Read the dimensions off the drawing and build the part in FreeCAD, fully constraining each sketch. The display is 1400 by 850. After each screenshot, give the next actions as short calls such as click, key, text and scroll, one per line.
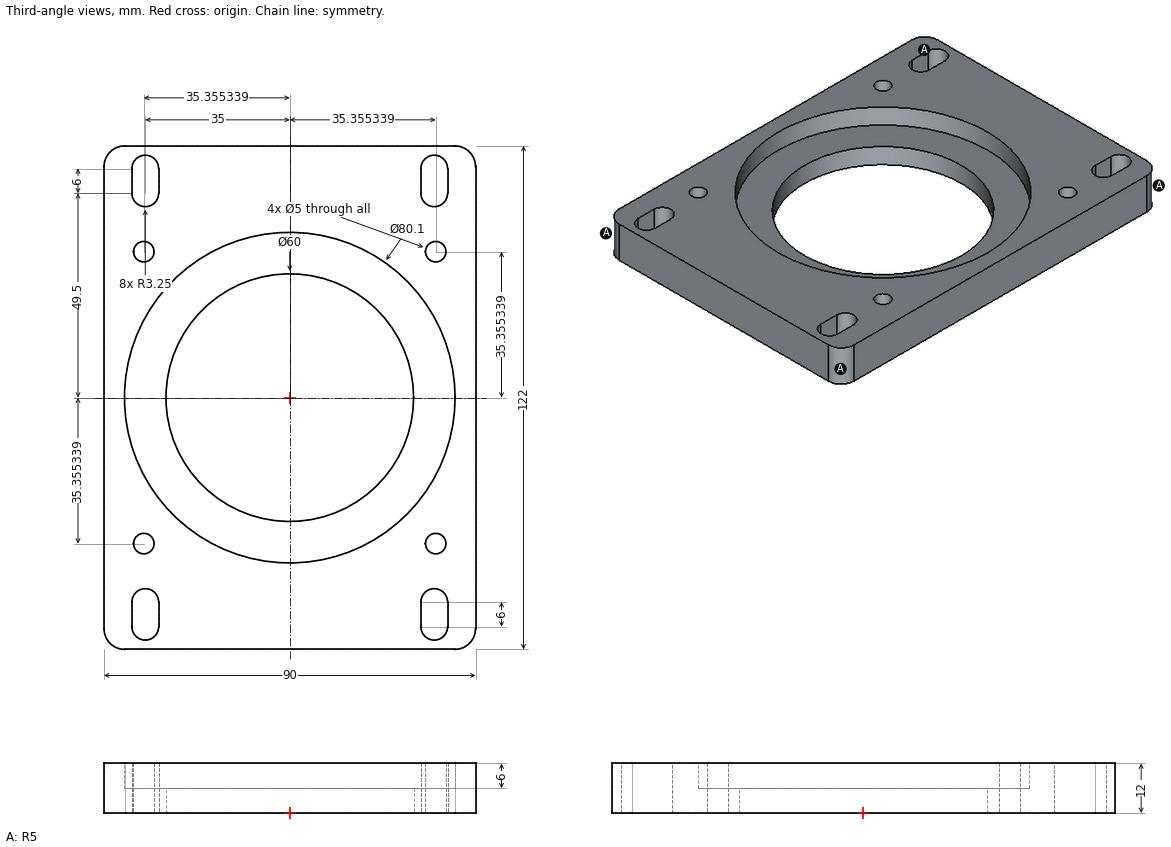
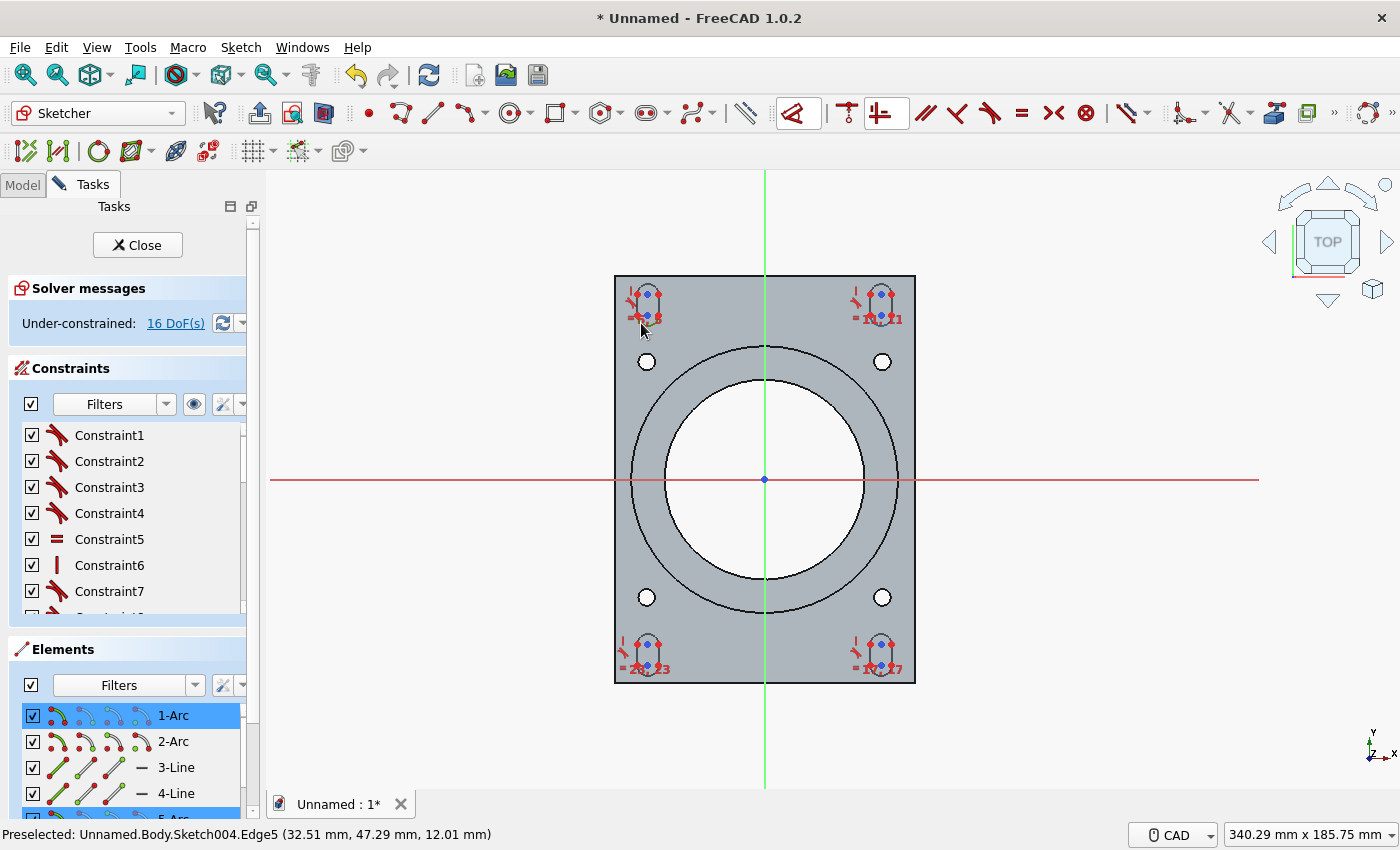
scroll(875, 674, up, 2)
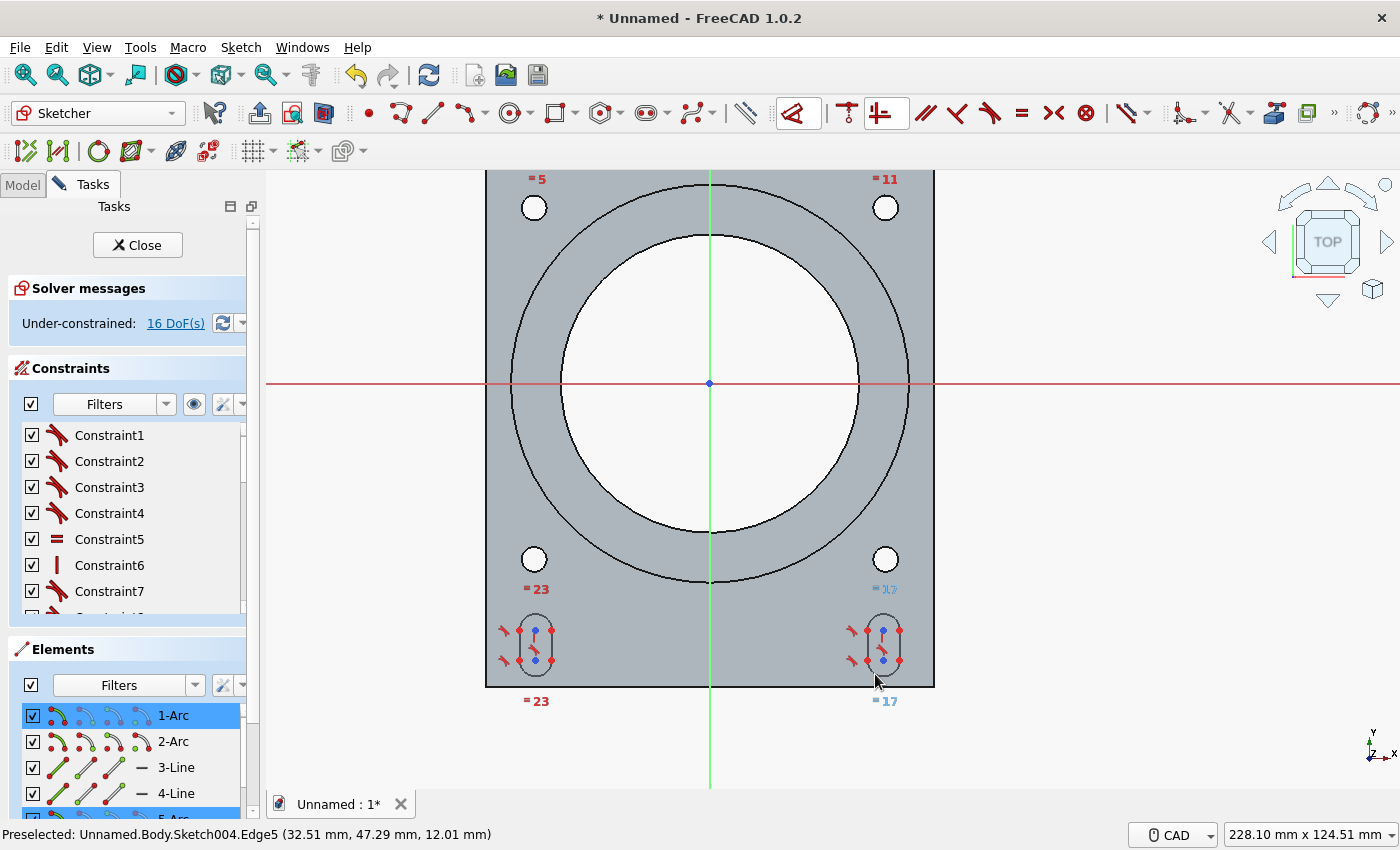
click(874, 673)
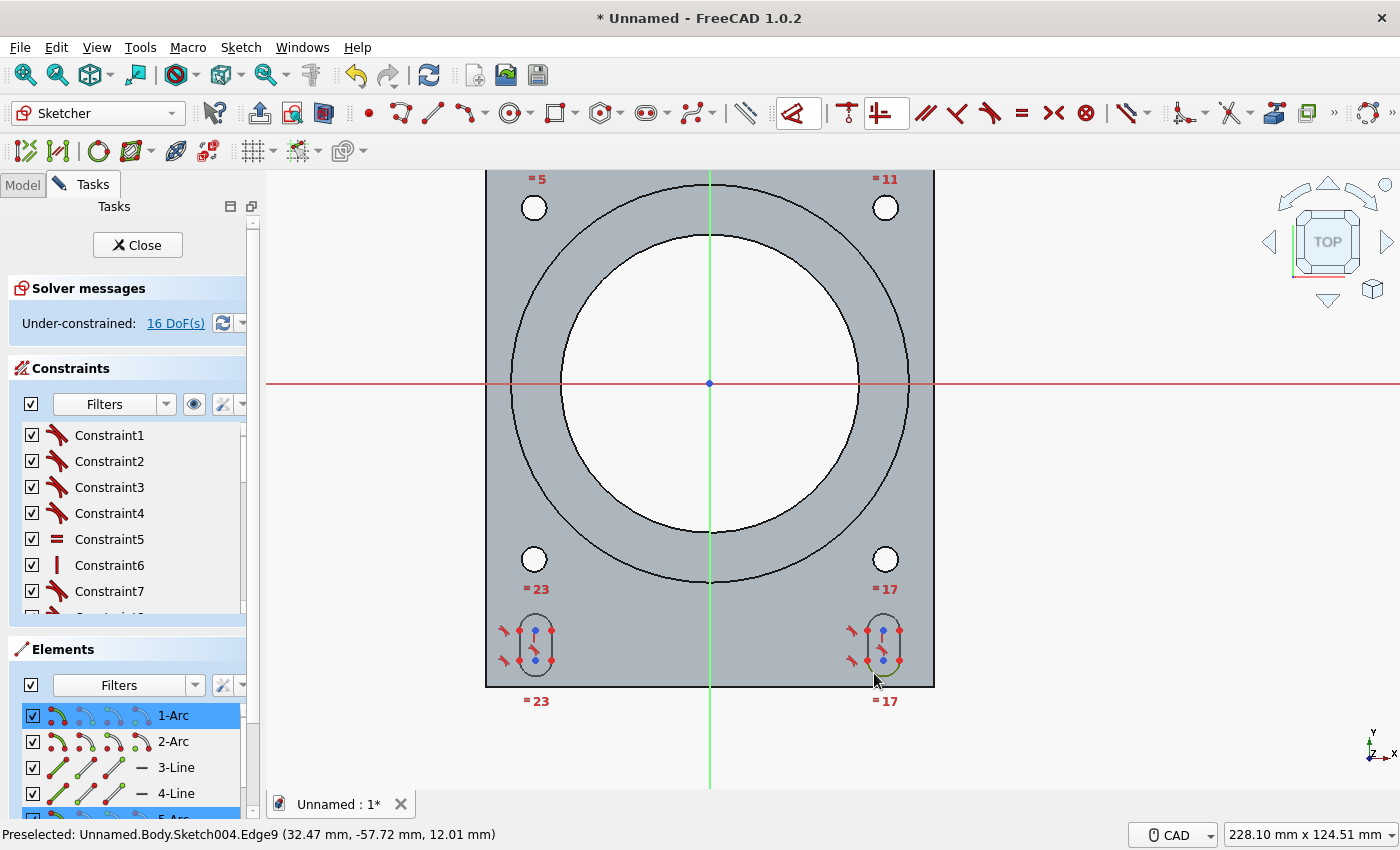
click(526, 673)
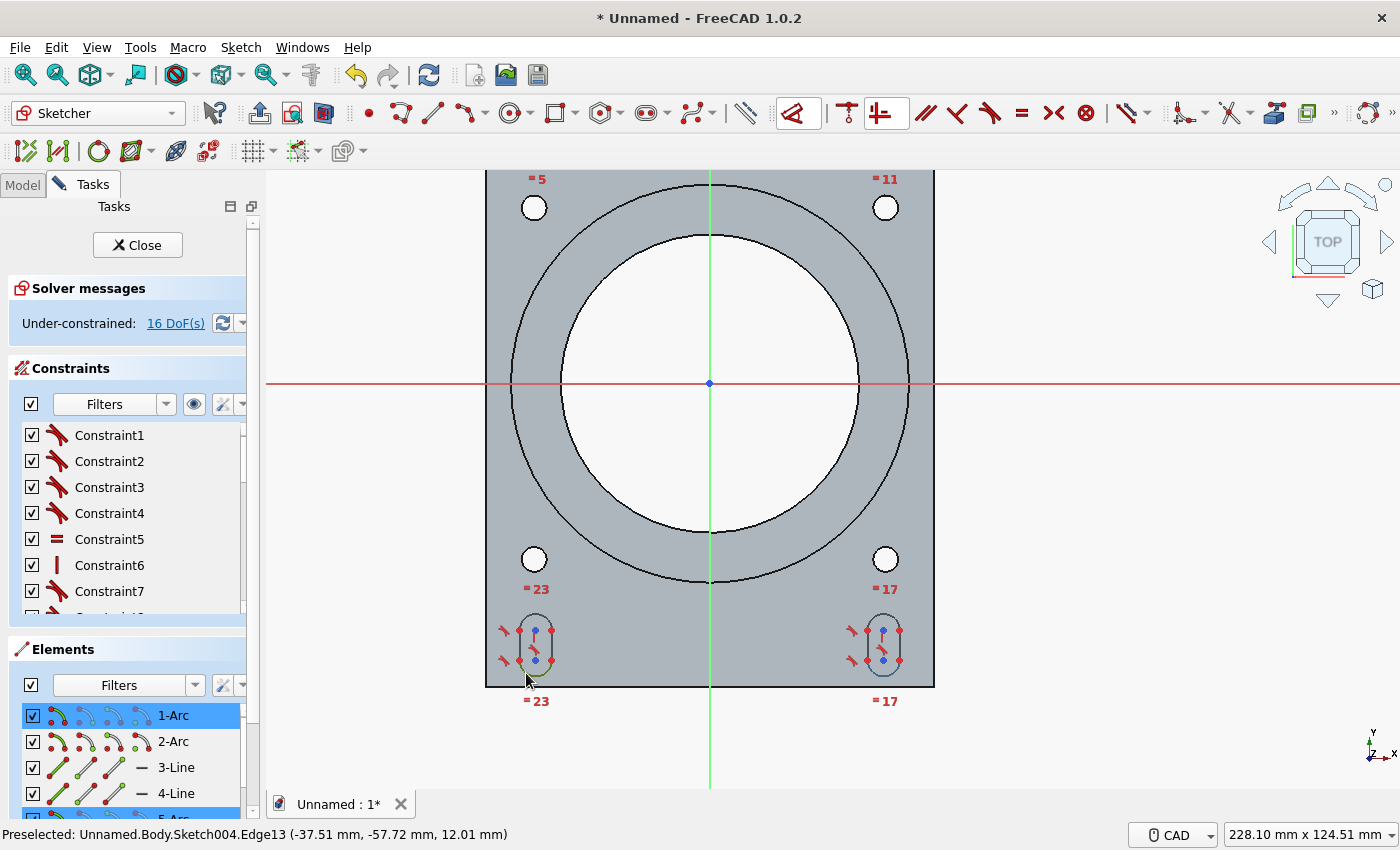
click(1022, 114)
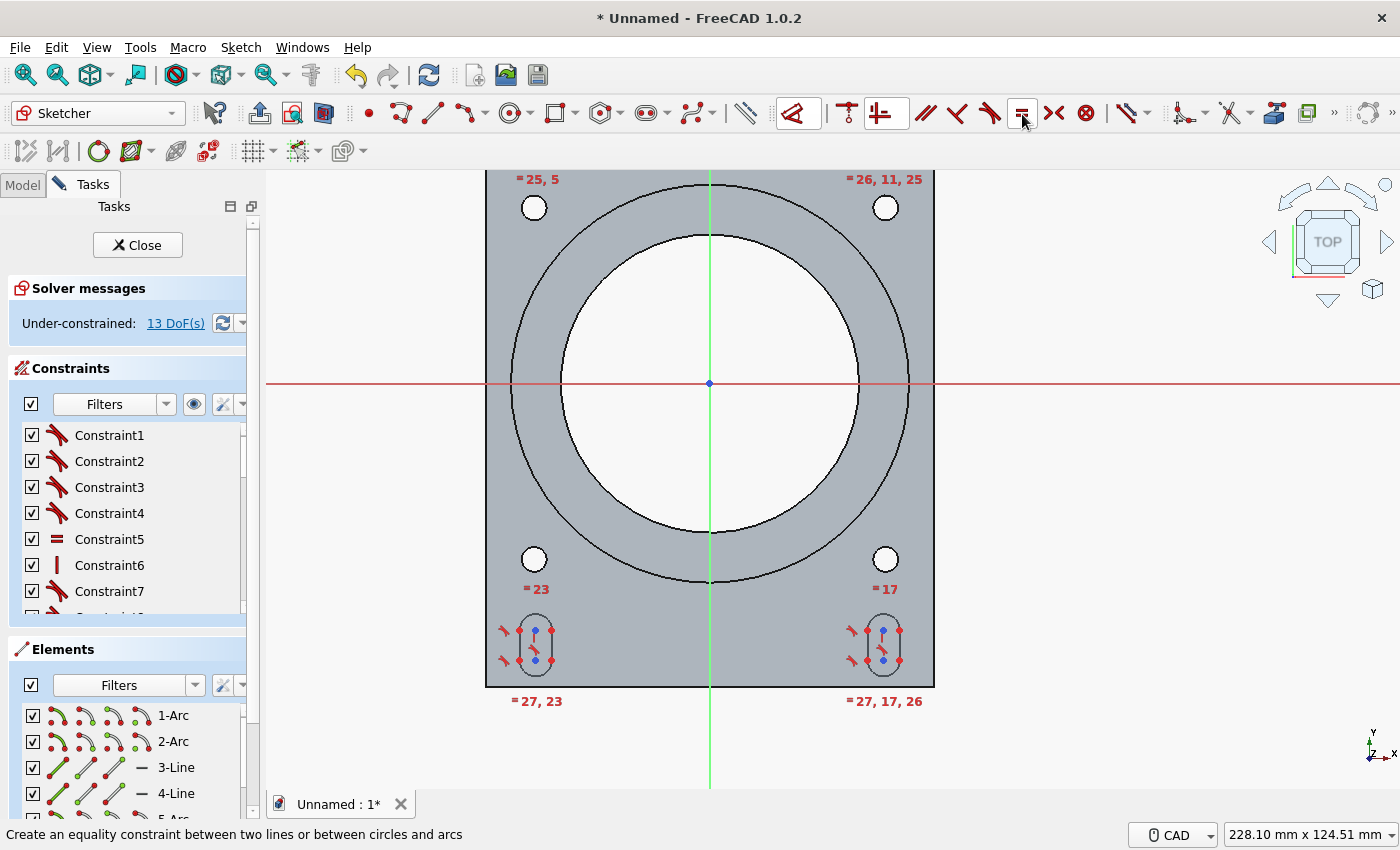
scroll(875, 674, down, 2)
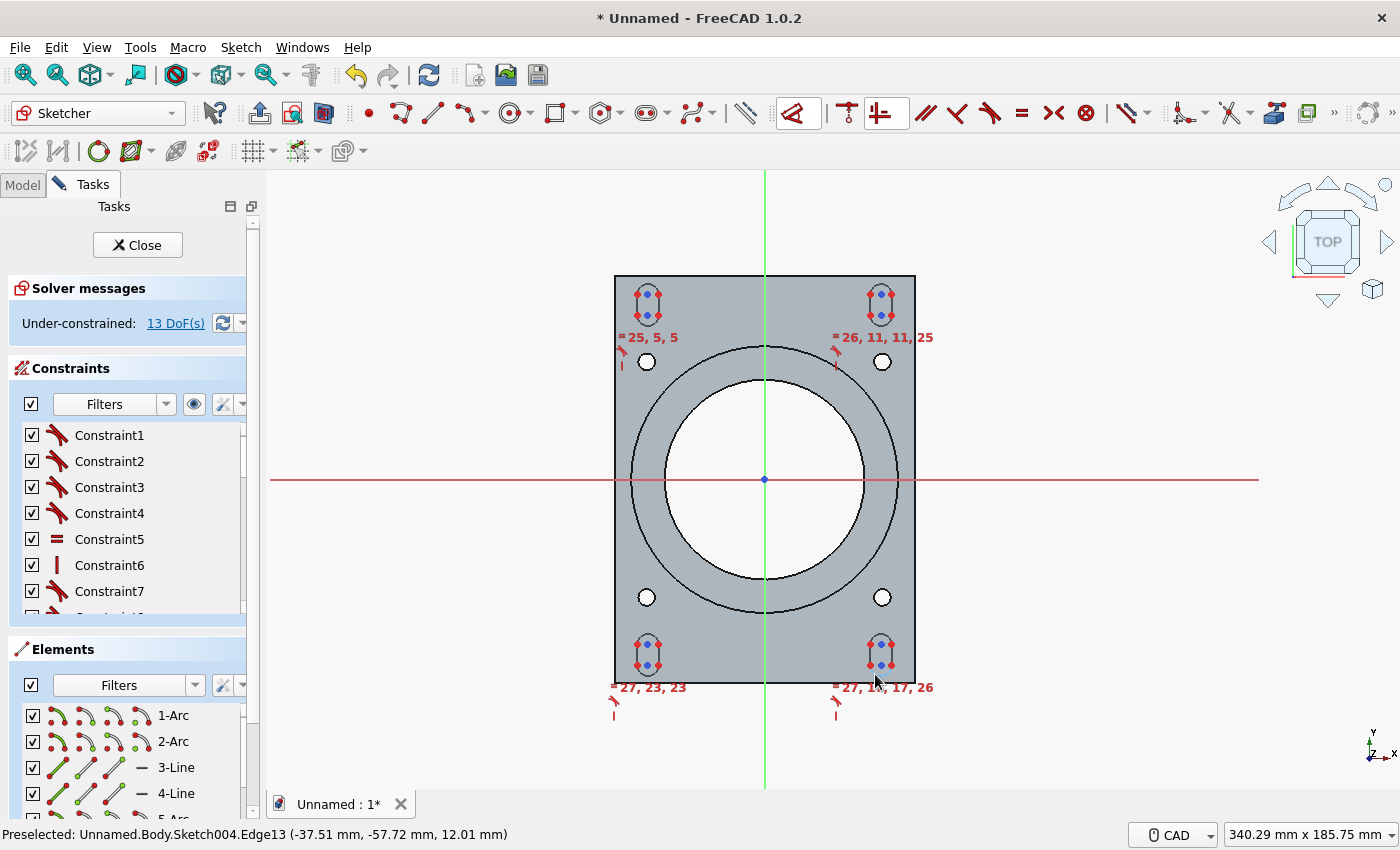
click(648, 315)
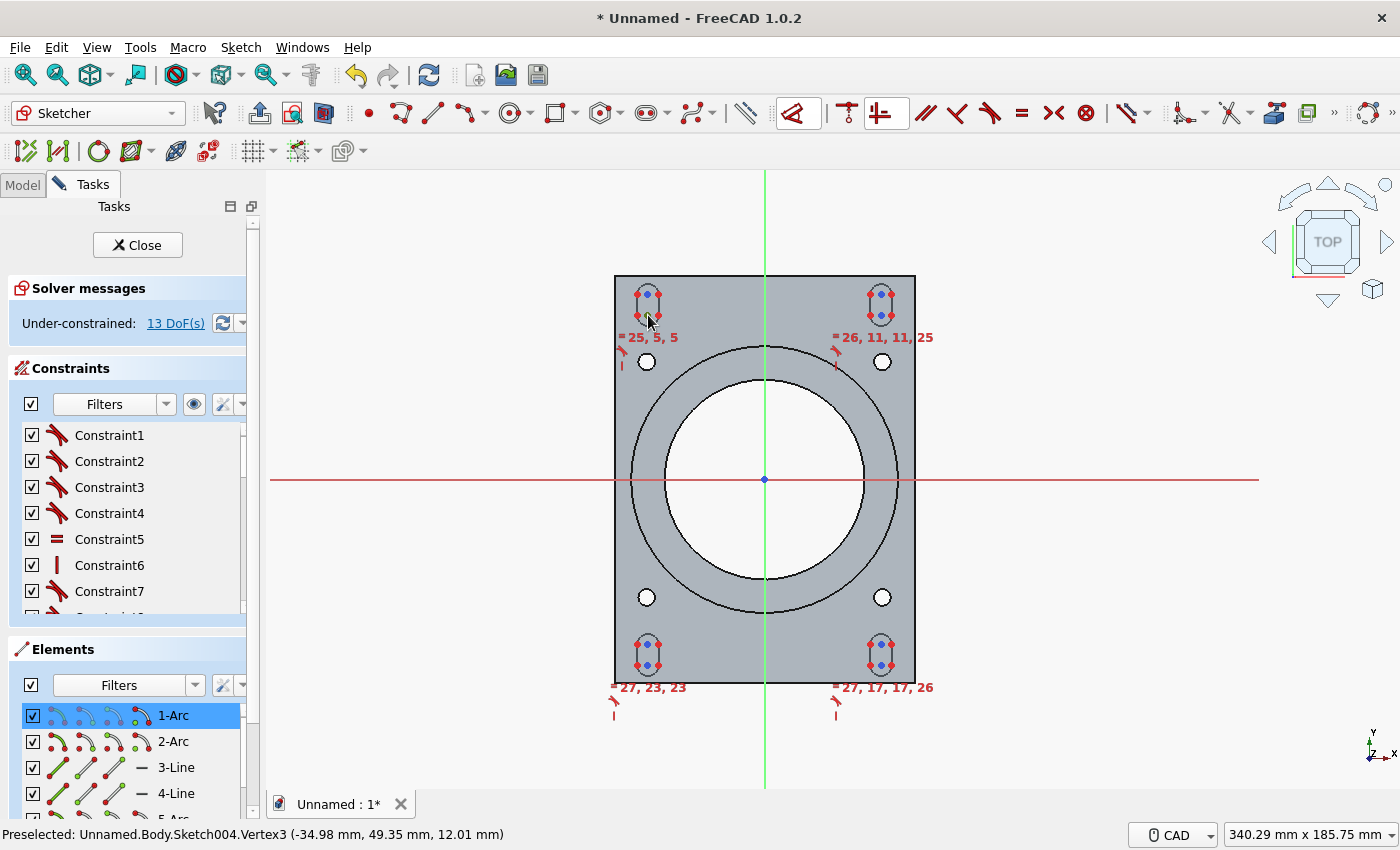
click(881, 315)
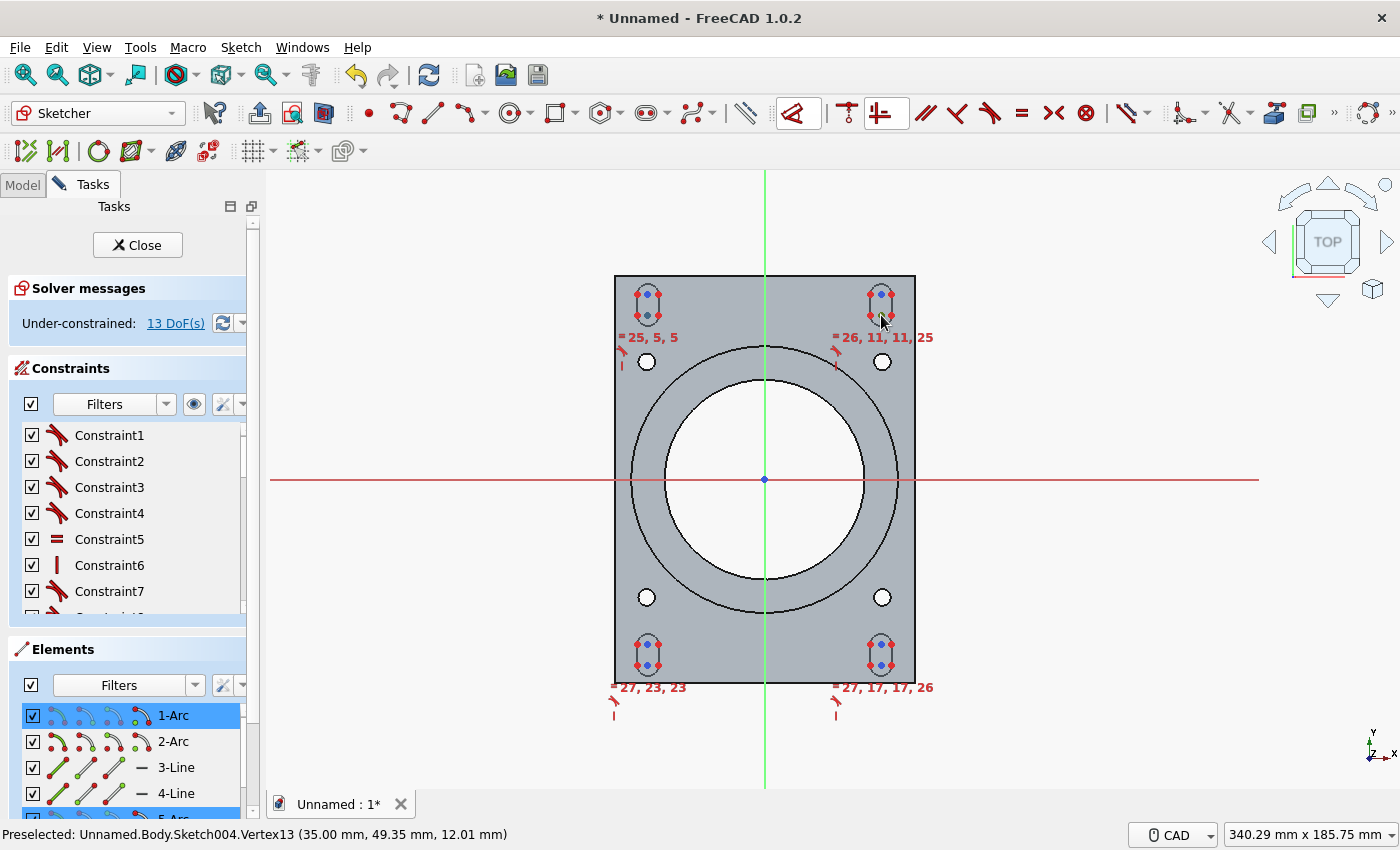
click(765, 721)